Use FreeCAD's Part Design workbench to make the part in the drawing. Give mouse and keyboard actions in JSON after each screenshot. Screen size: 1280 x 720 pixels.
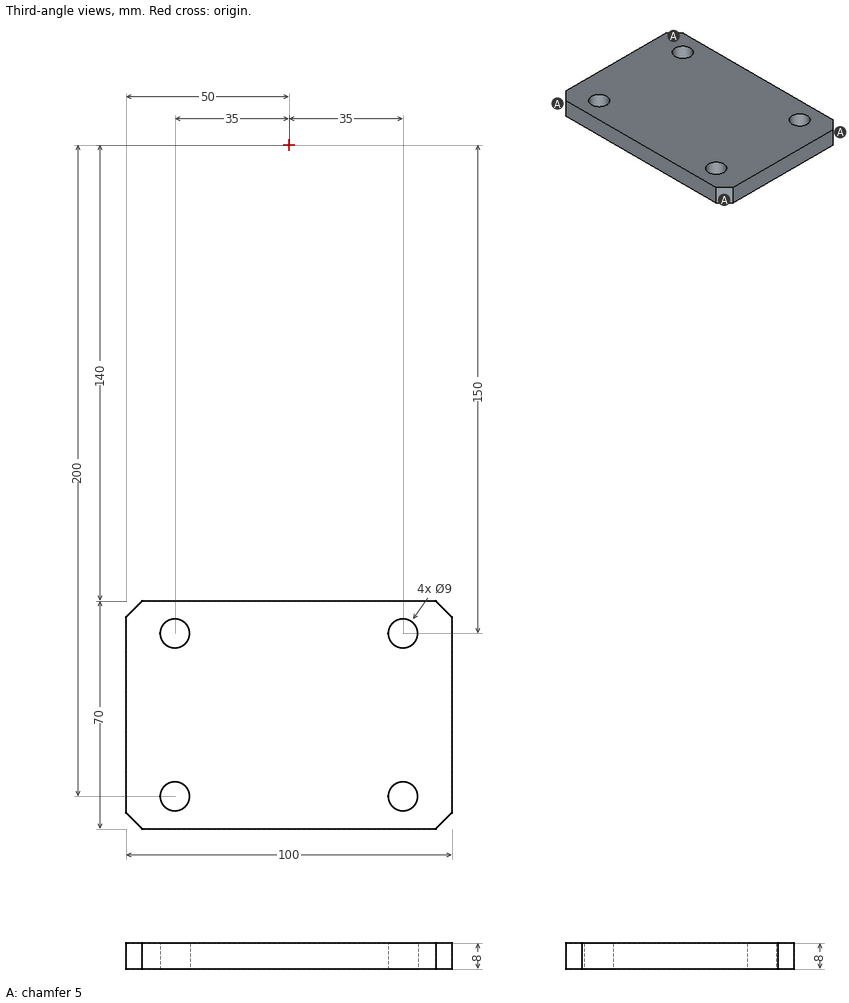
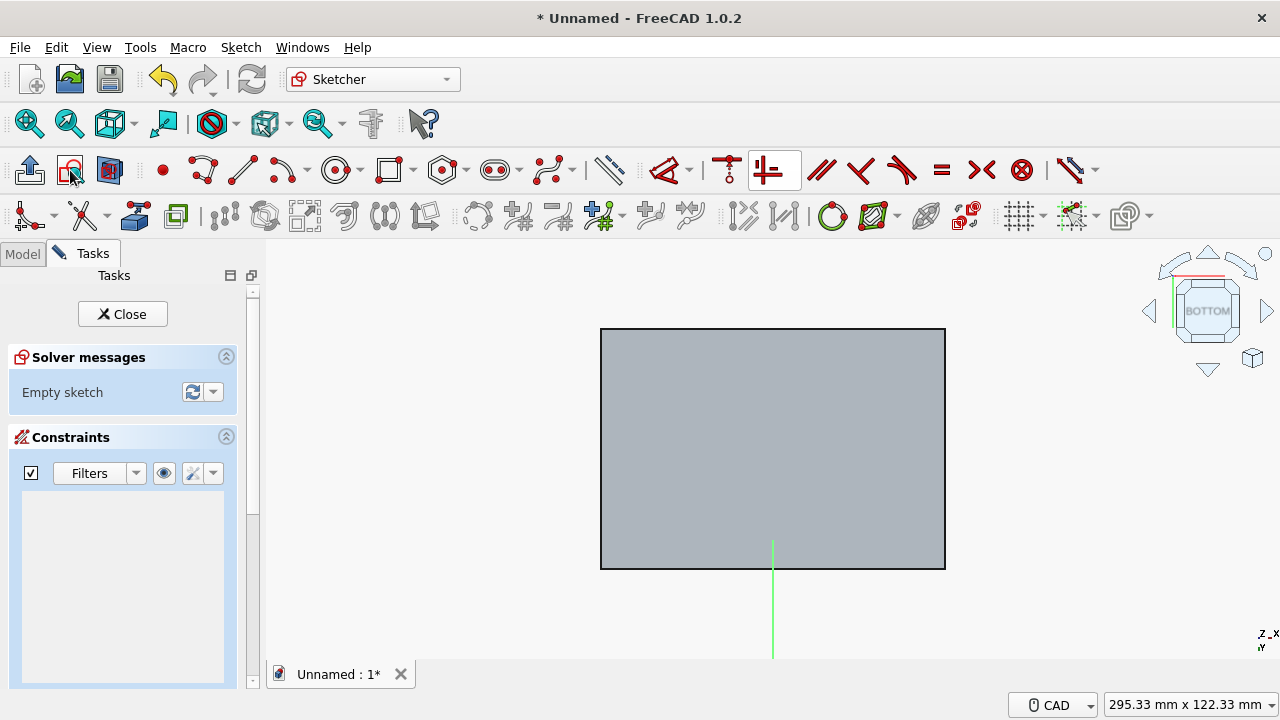
{"action": "left_click", "coordinate": [336, 170]}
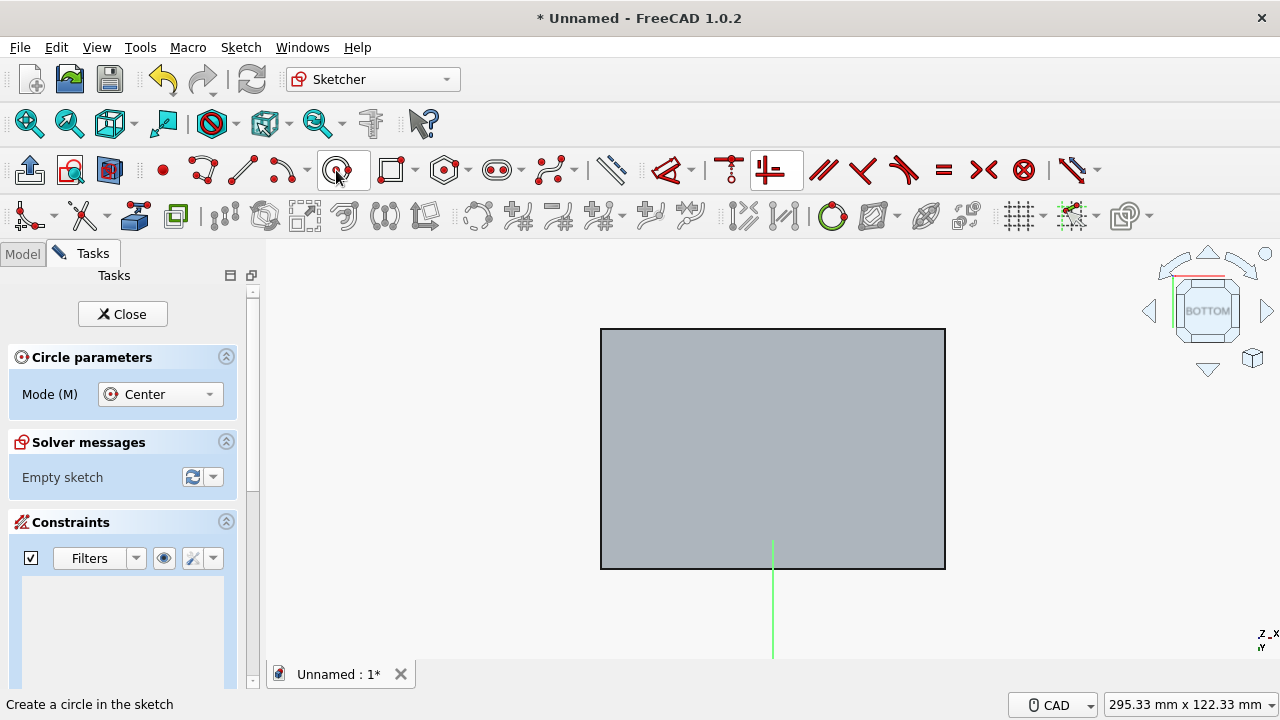
{"action": "scroll", "coordinate": [893, 535], "scroll_direction": "up", "scroll_amount": 2}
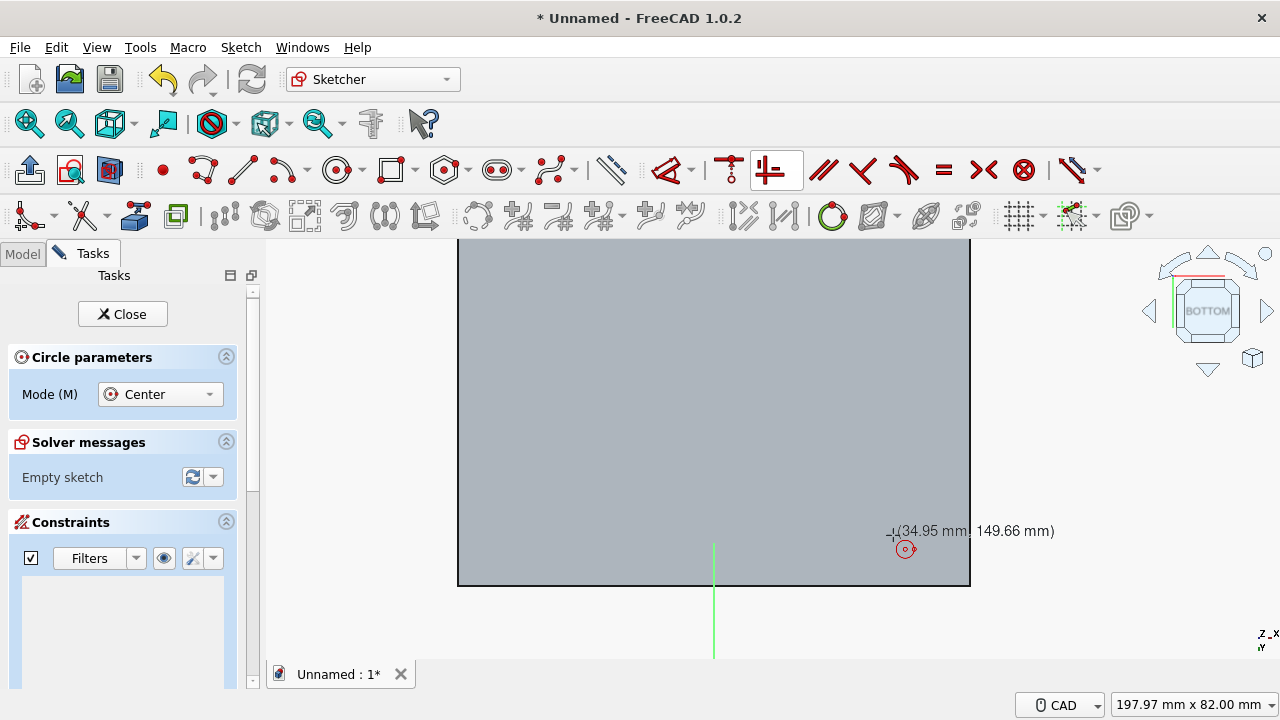
{"action": "left_click", "coordinate": [893, 534]}
{"action": "left_click", "coordinate": [909, 518]}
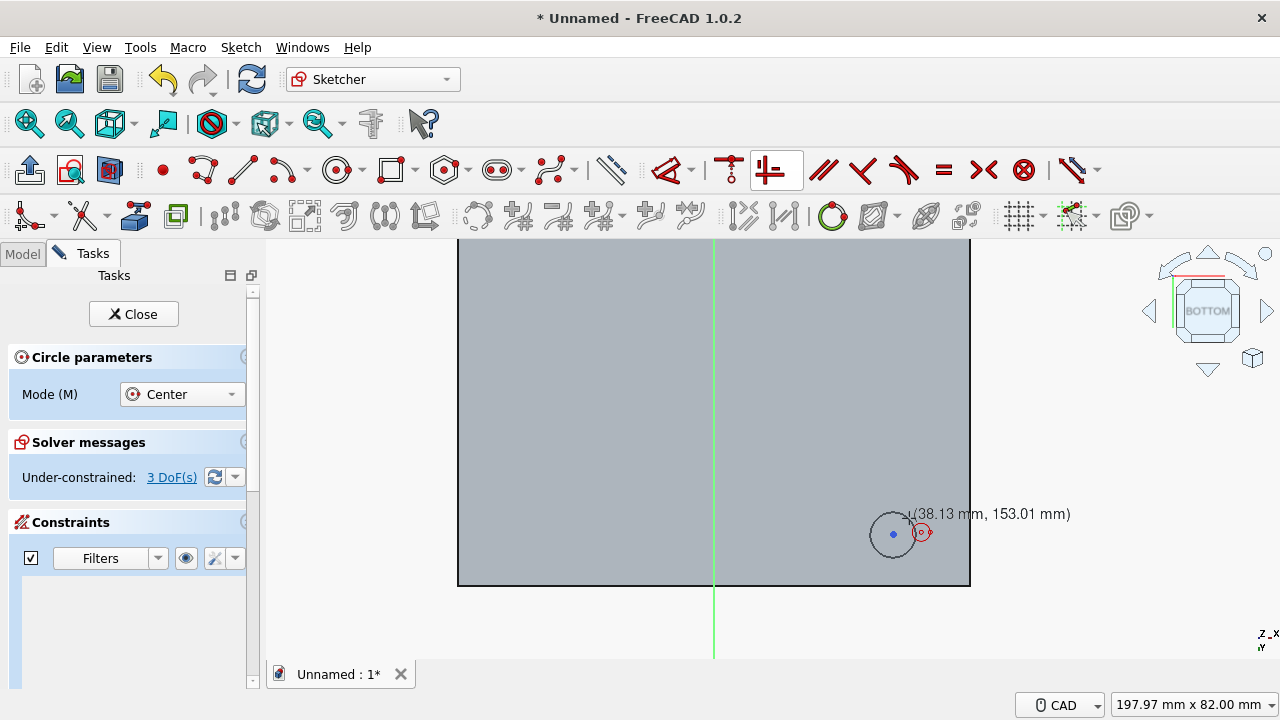
{"action": "left_click", "coordinate": [534, 534]}
{"action": "left_click", "coordinate": [551, 518]}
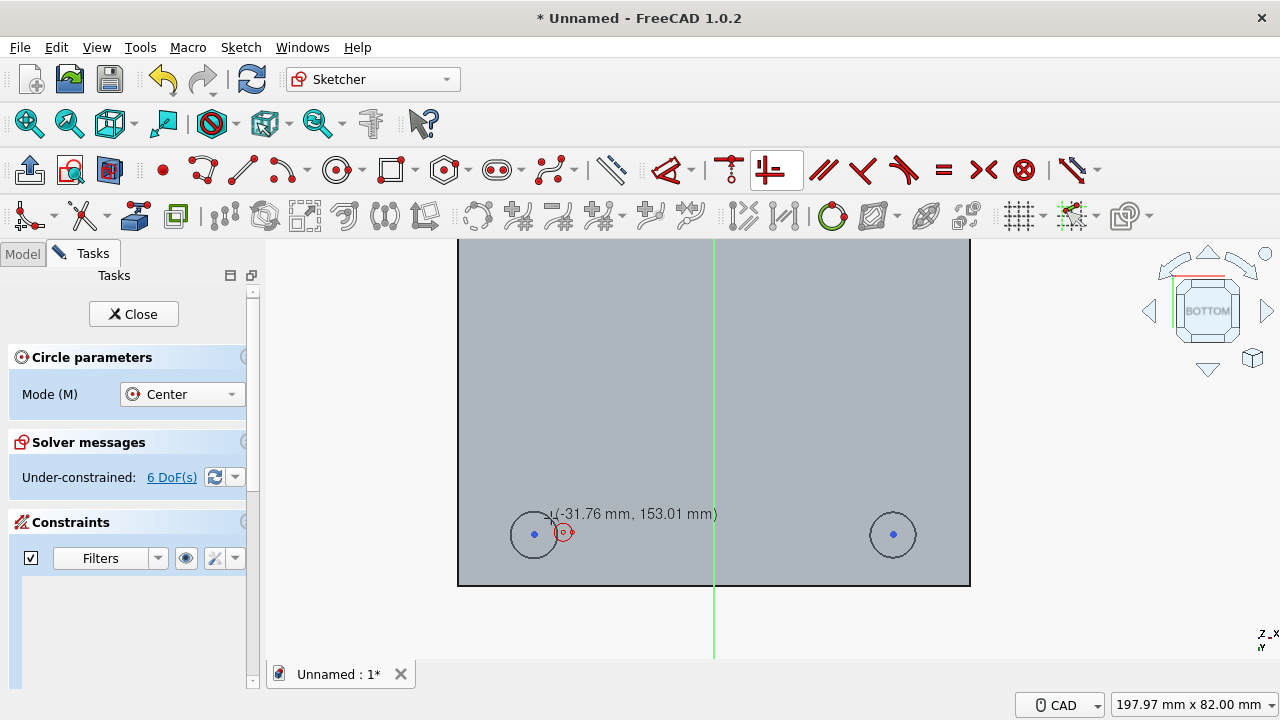
{"action": "left_click", "coordinate": [534, 278]}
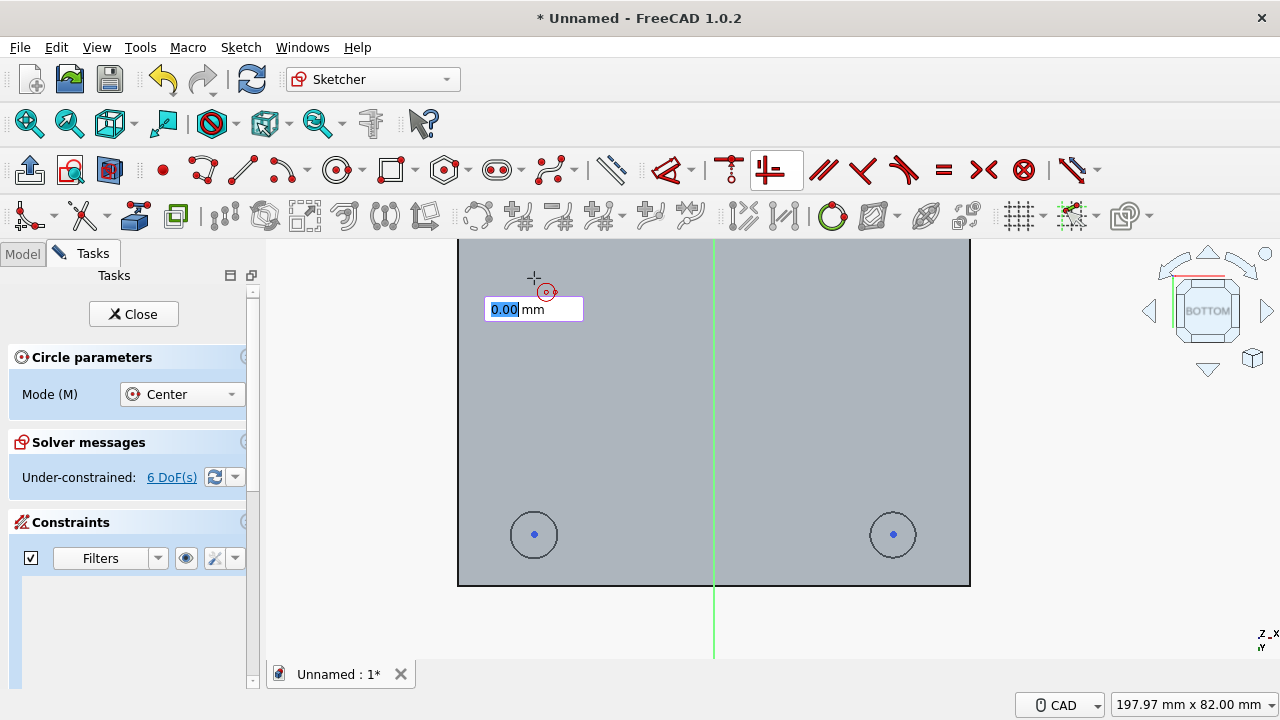
{"action": "scroll", "coordinate": [663, 631], "scroll_direction": "down", "scroll_amount": 1}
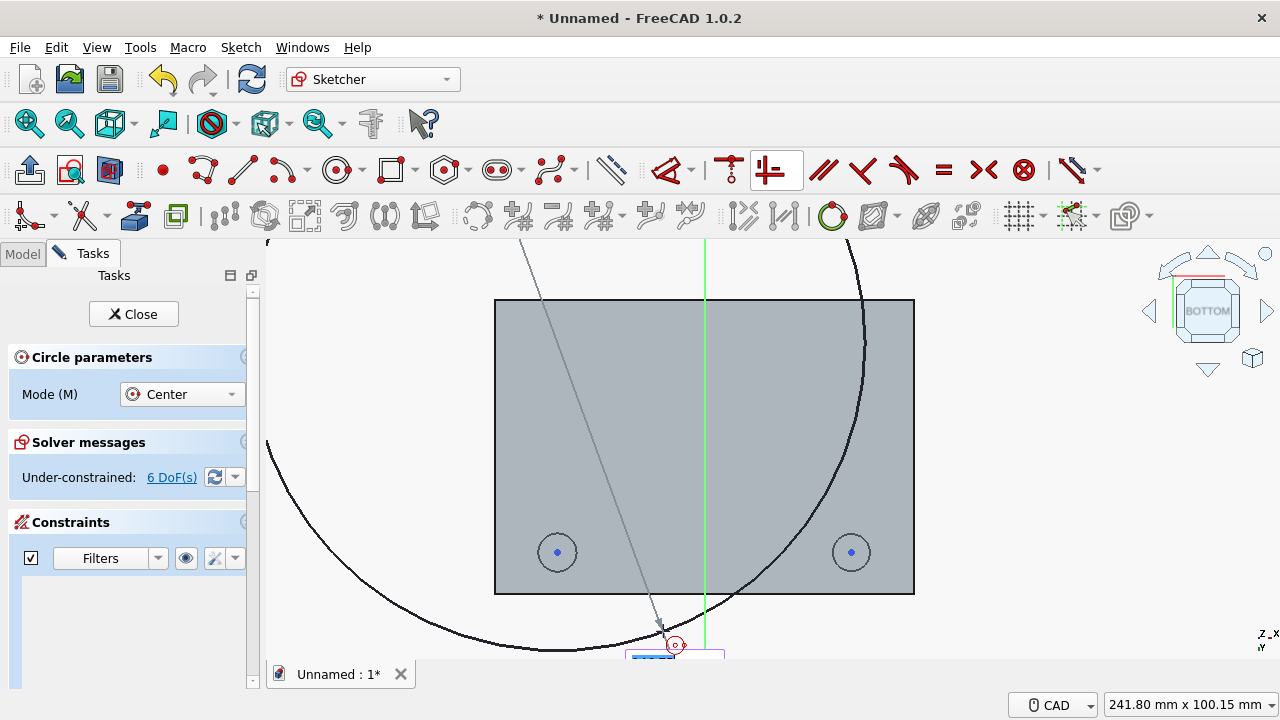
{"action": "left_click", "coordinate": [571, 329]}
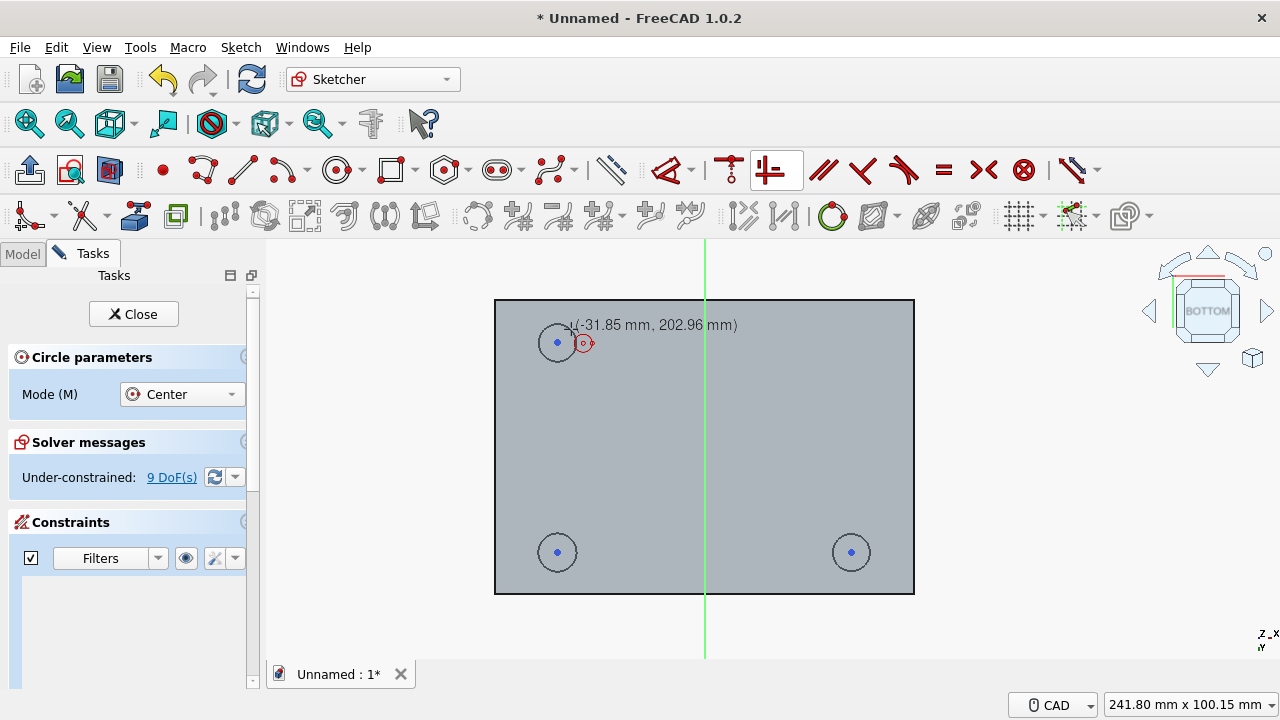
{"action": "left_click", "coordinate": [851, 342]}
{"action": "left_click", "coordinate": [865, 329]}
{"action": "key", "text": "Escape"}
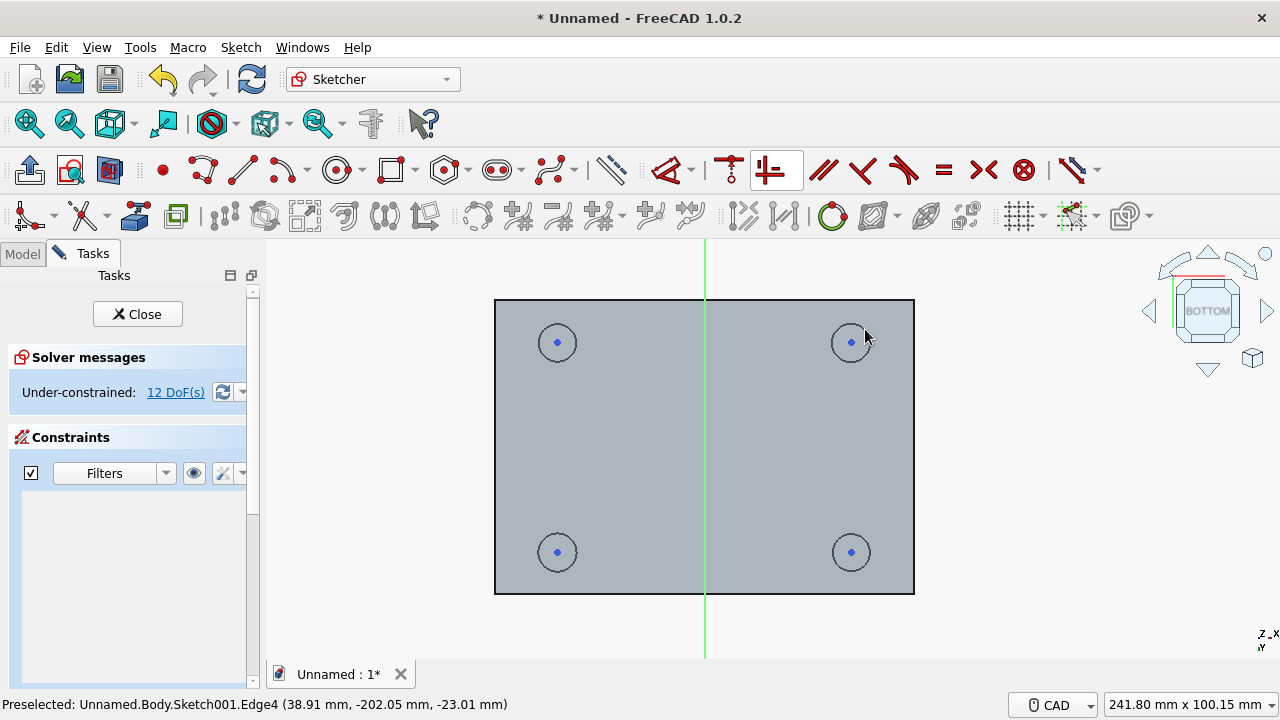
{"action": "left_click", "coordinate": [864, 539]}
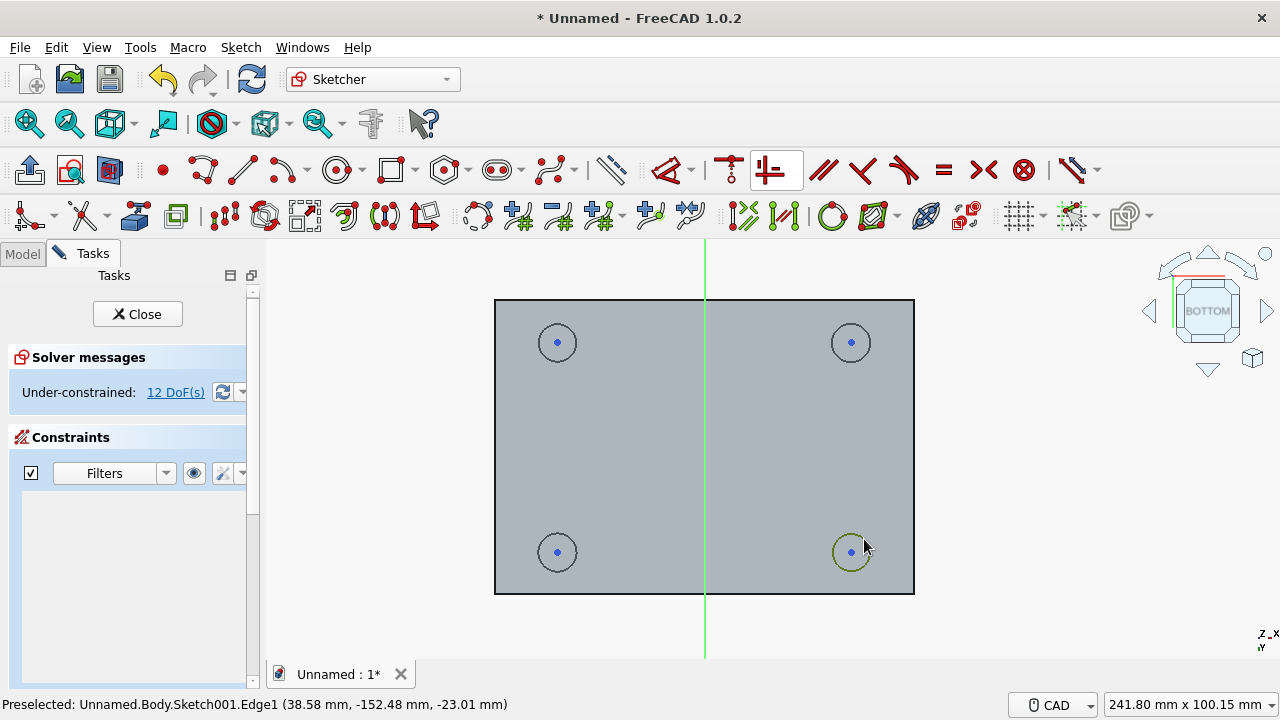
{"action": "left_click", "coordinate": [571, 539]}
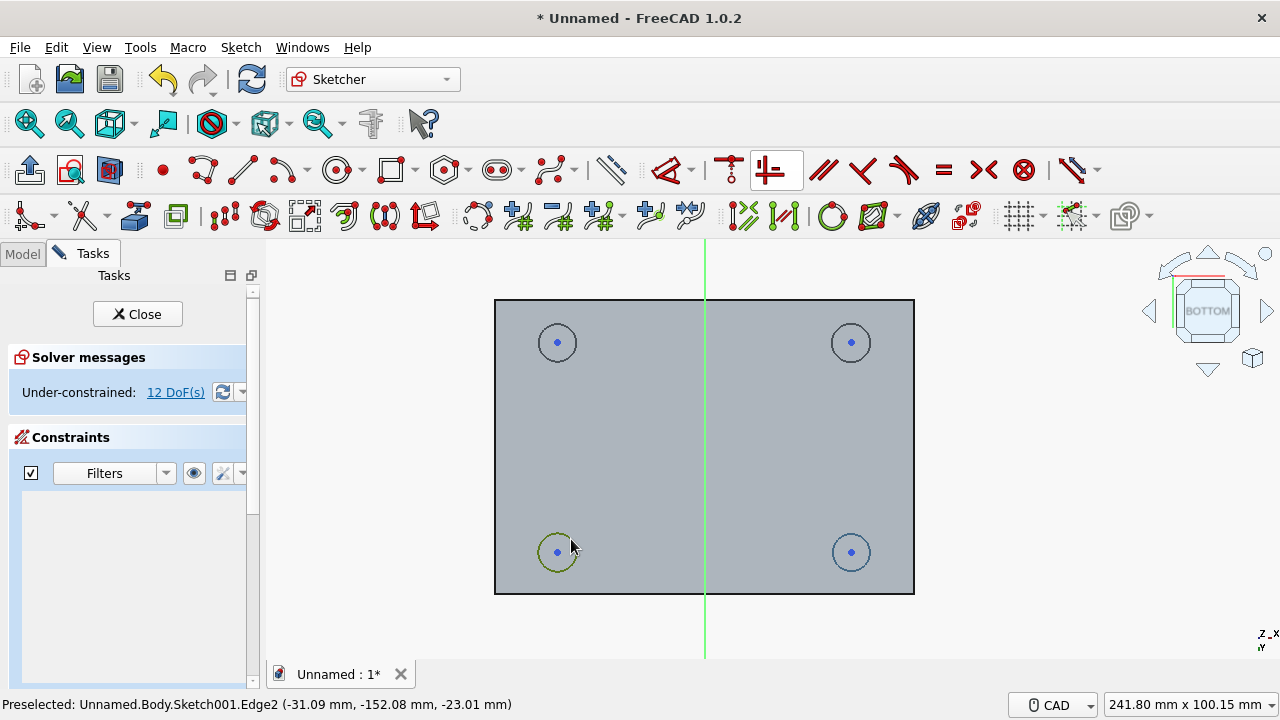
{"action": "left_click", "coordinate": [571, 330]}